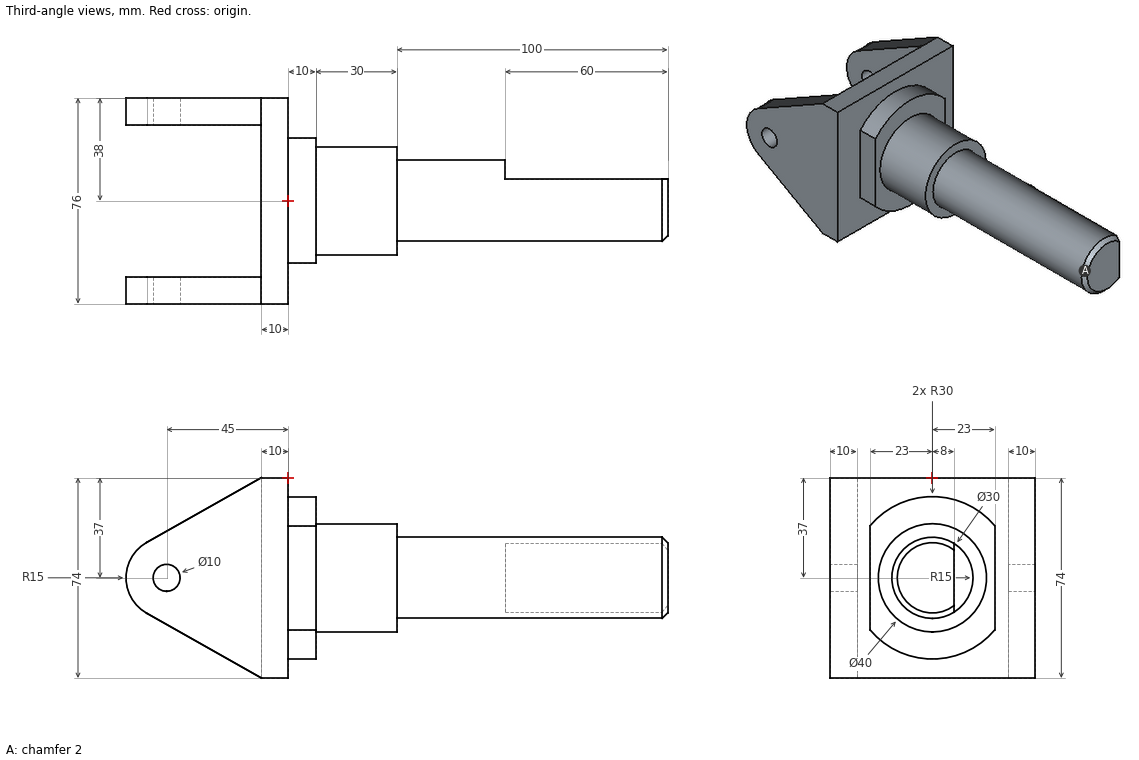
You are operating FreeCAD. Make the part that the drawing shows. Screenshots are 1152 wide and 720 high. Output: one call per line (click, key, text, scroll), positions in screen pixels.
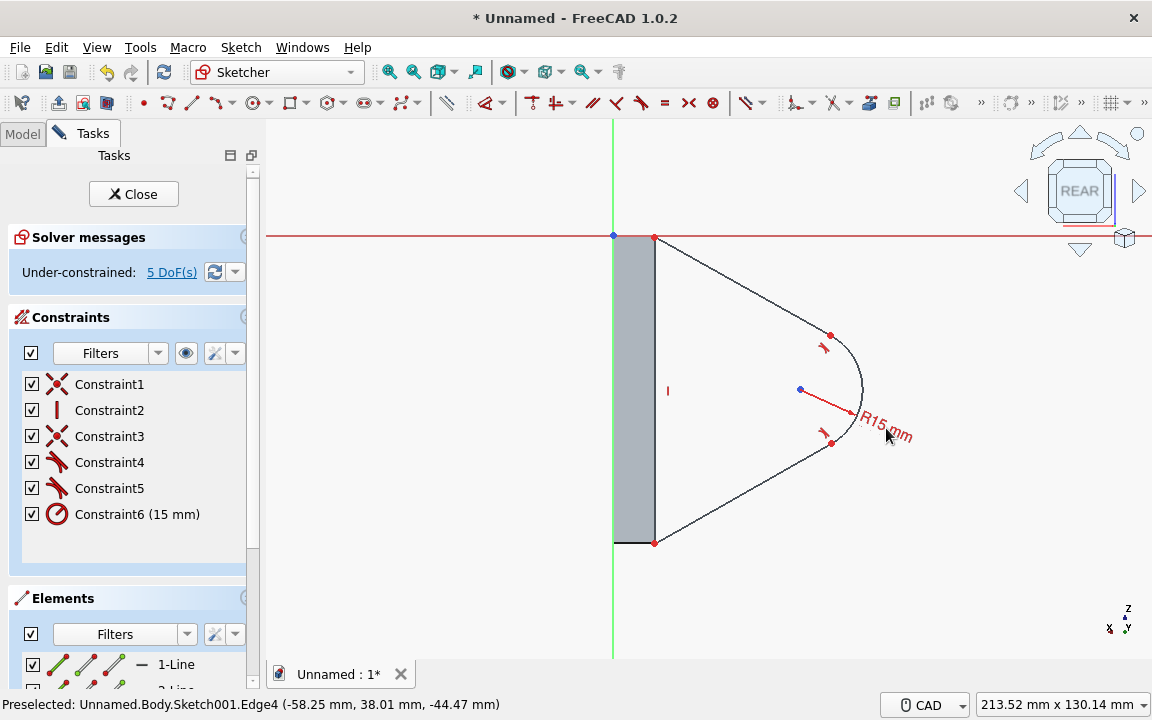
click(655, 237)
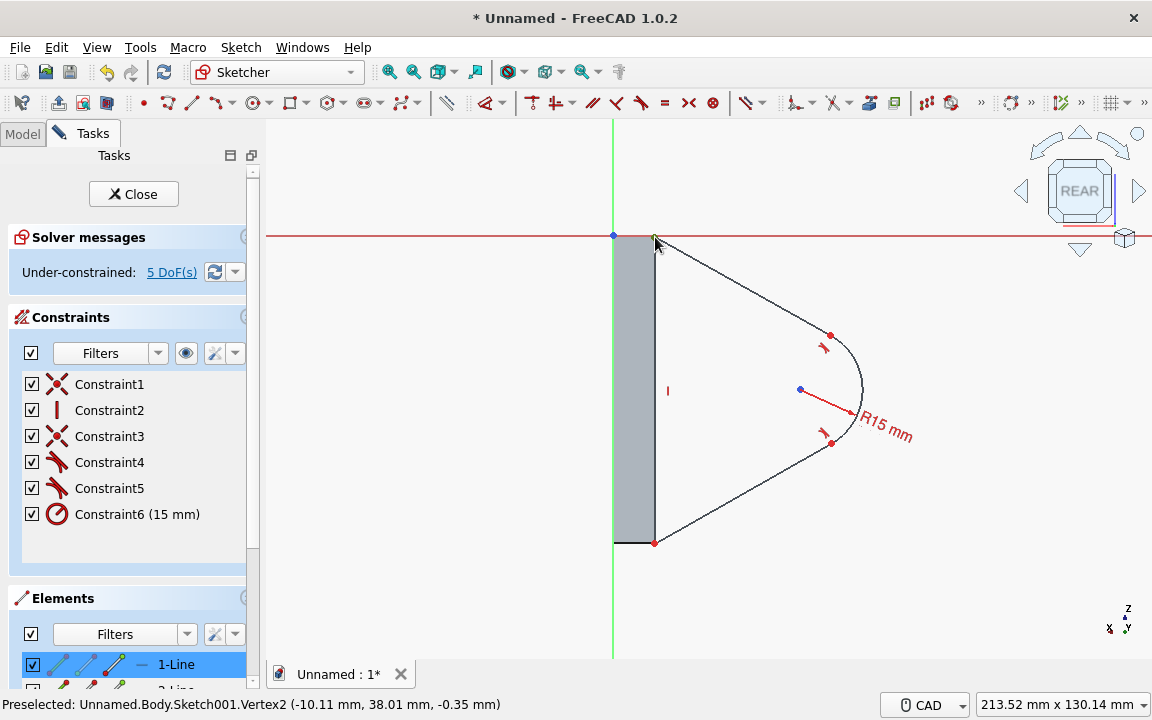
click(344, 236)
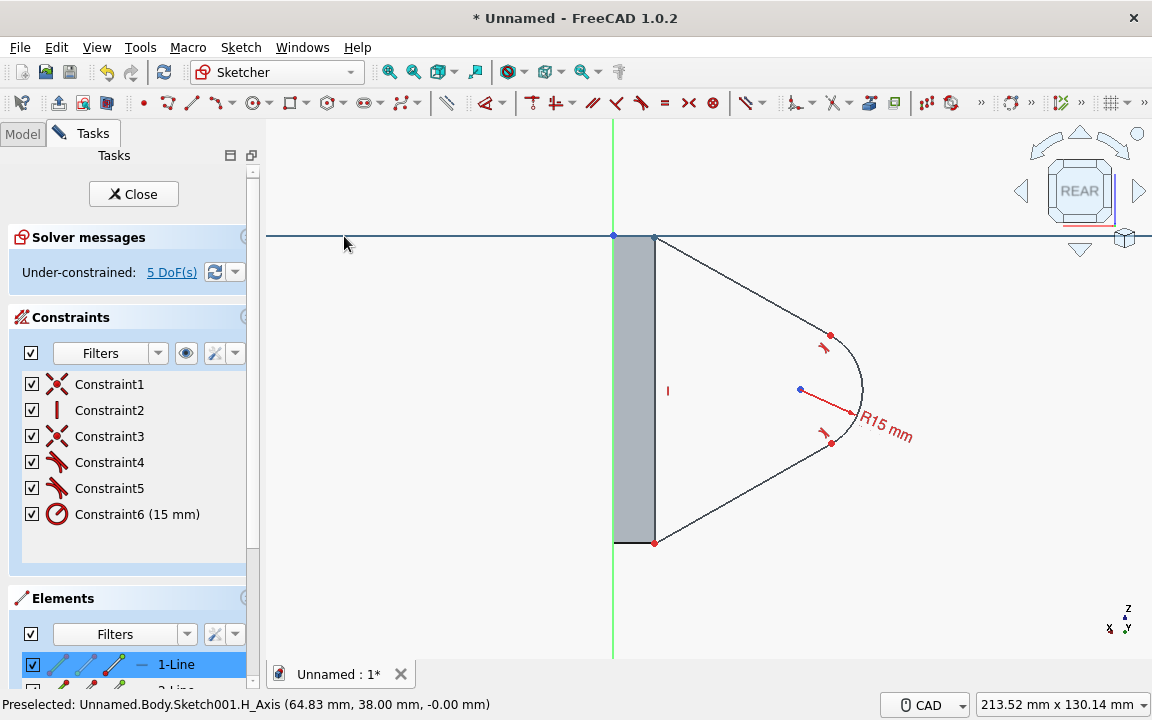
click(532, 104)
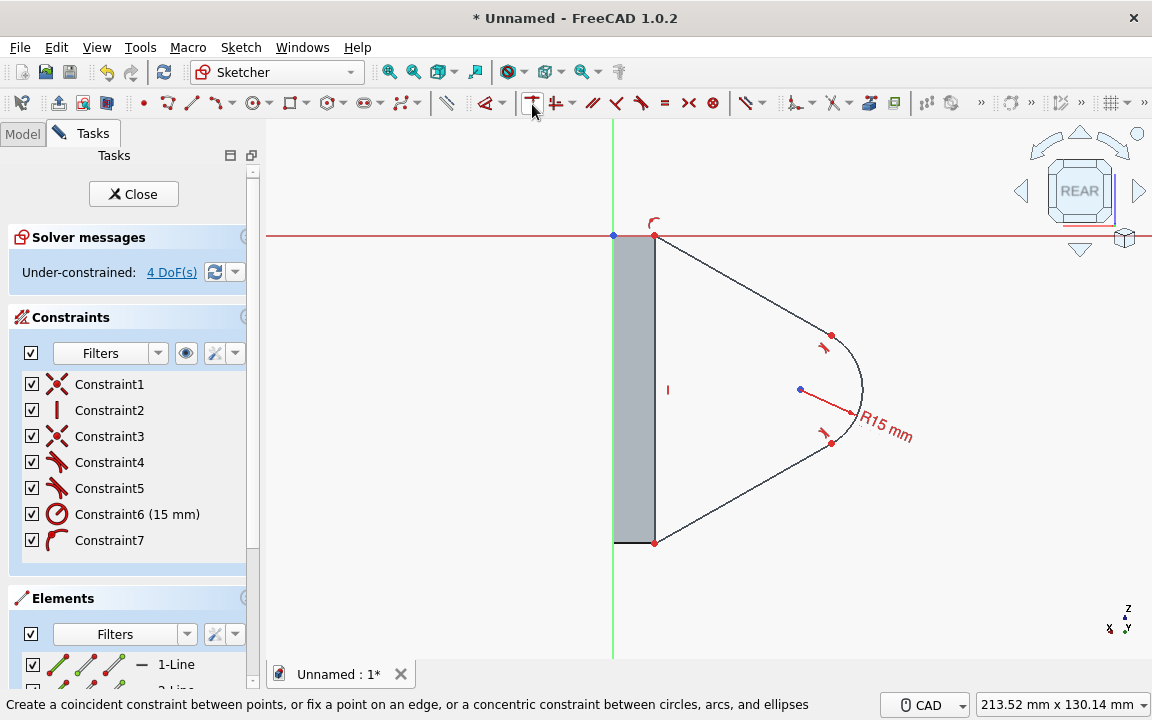
click(486, 104)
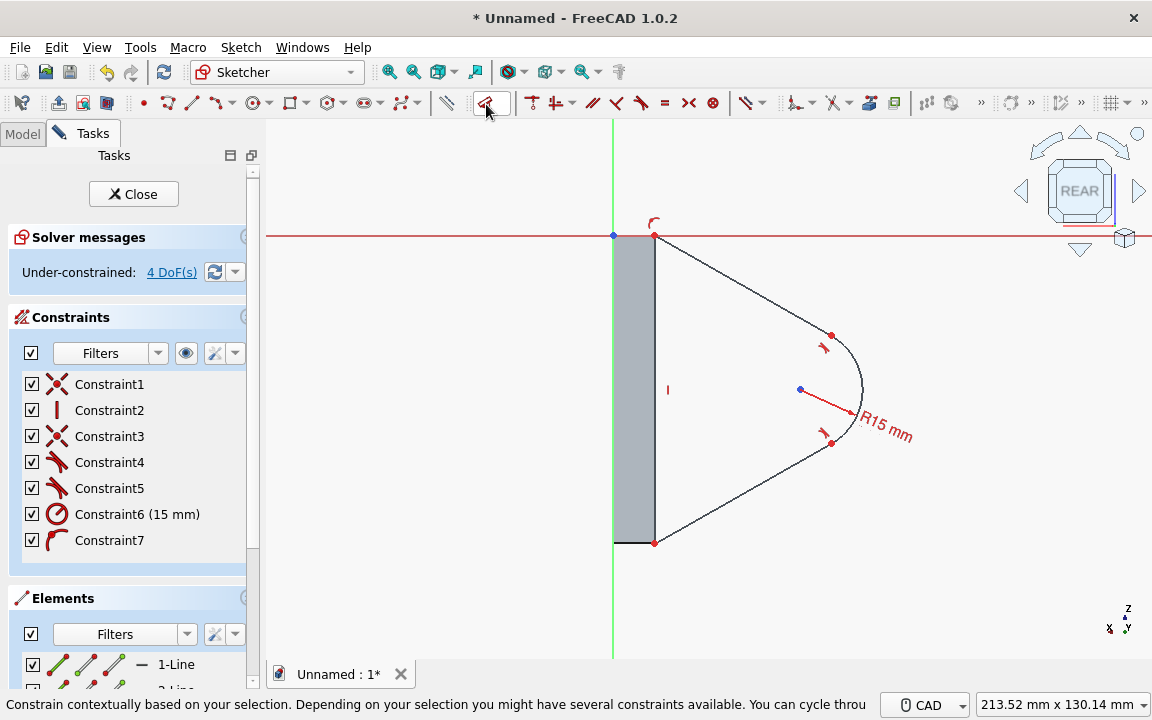
click(655, 328)
click(689, 390)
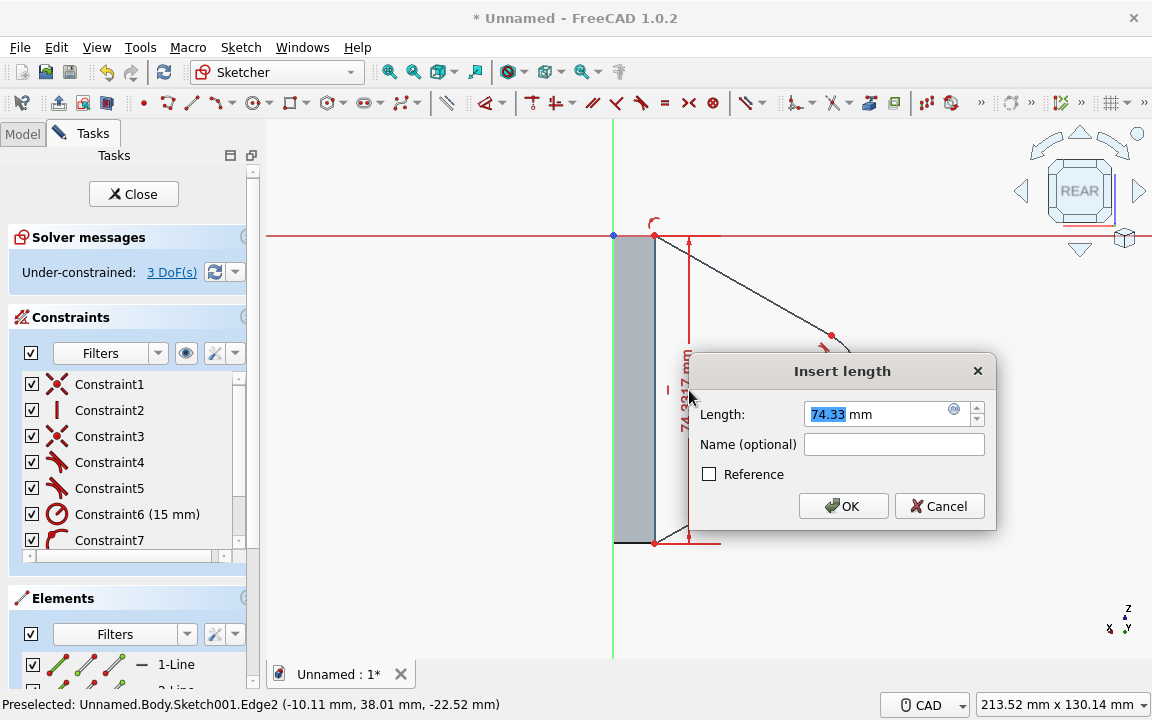
text(74)
key(Return)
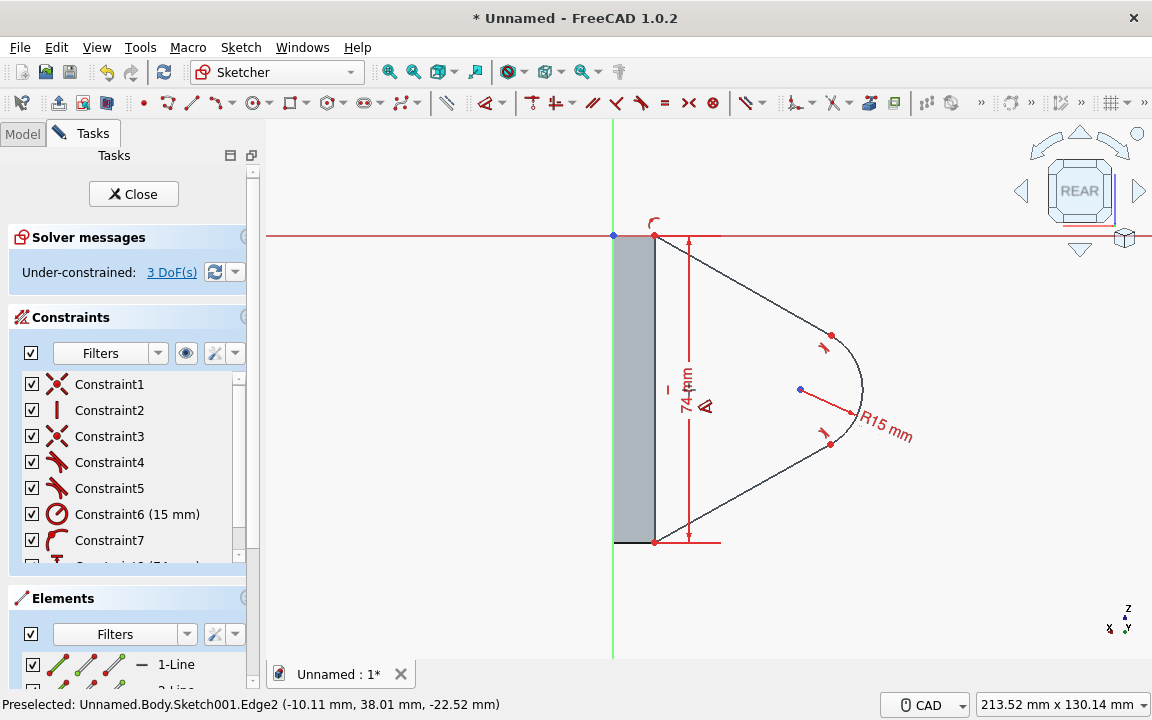
click(655, 236)
click(634, 202)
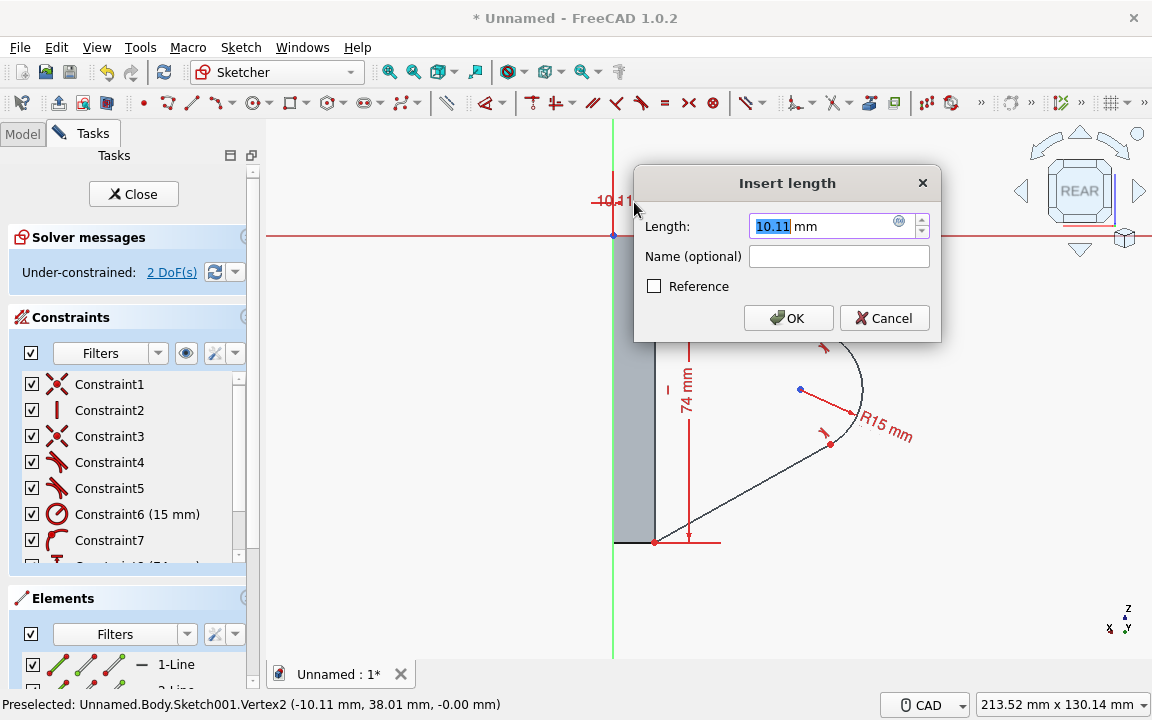
text(10)
key(Return)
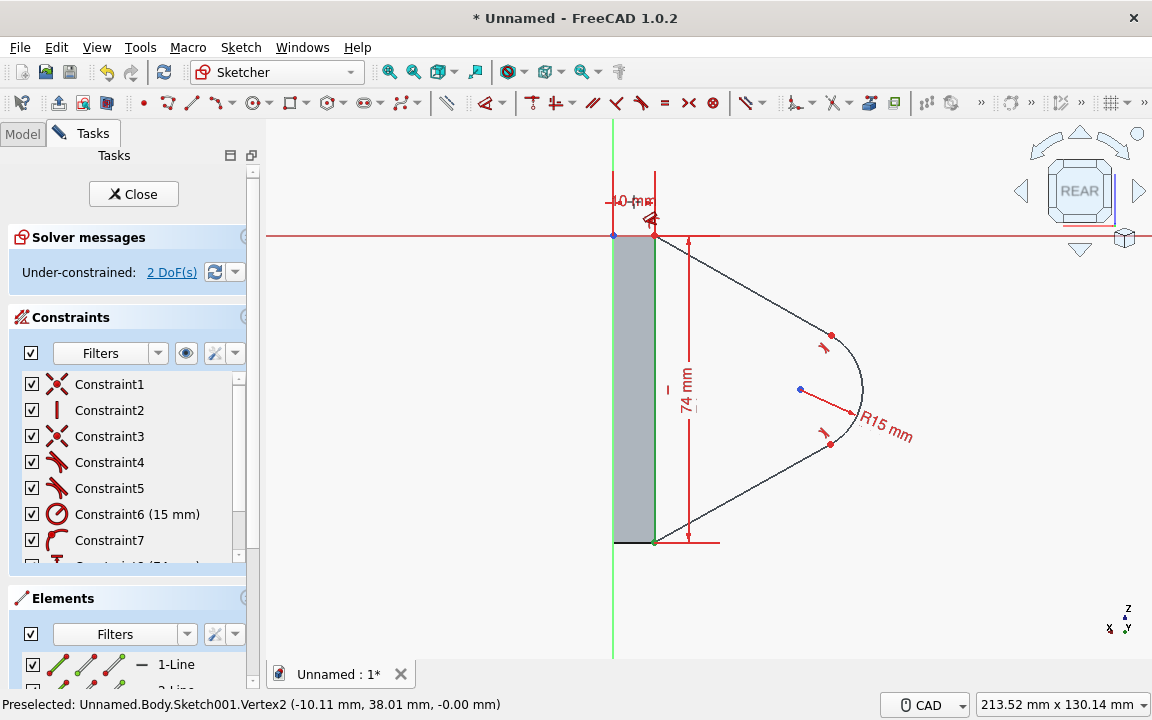
click(800, 390)
click(707, 202)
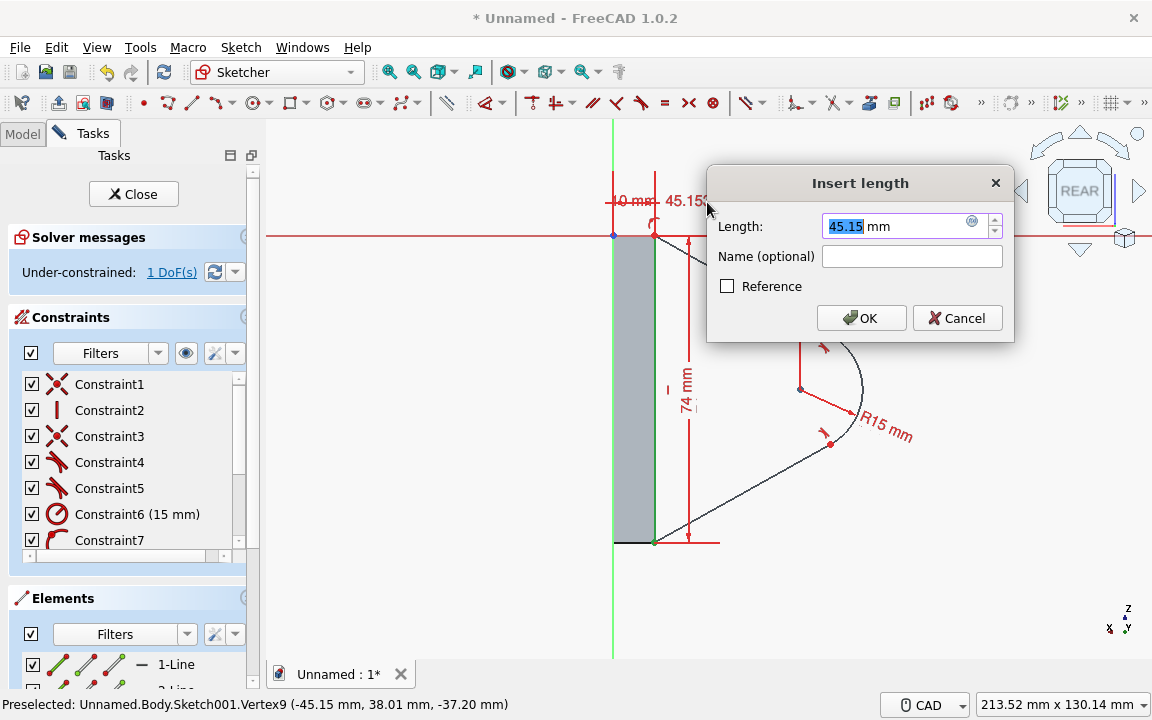
text(45)
key(Return)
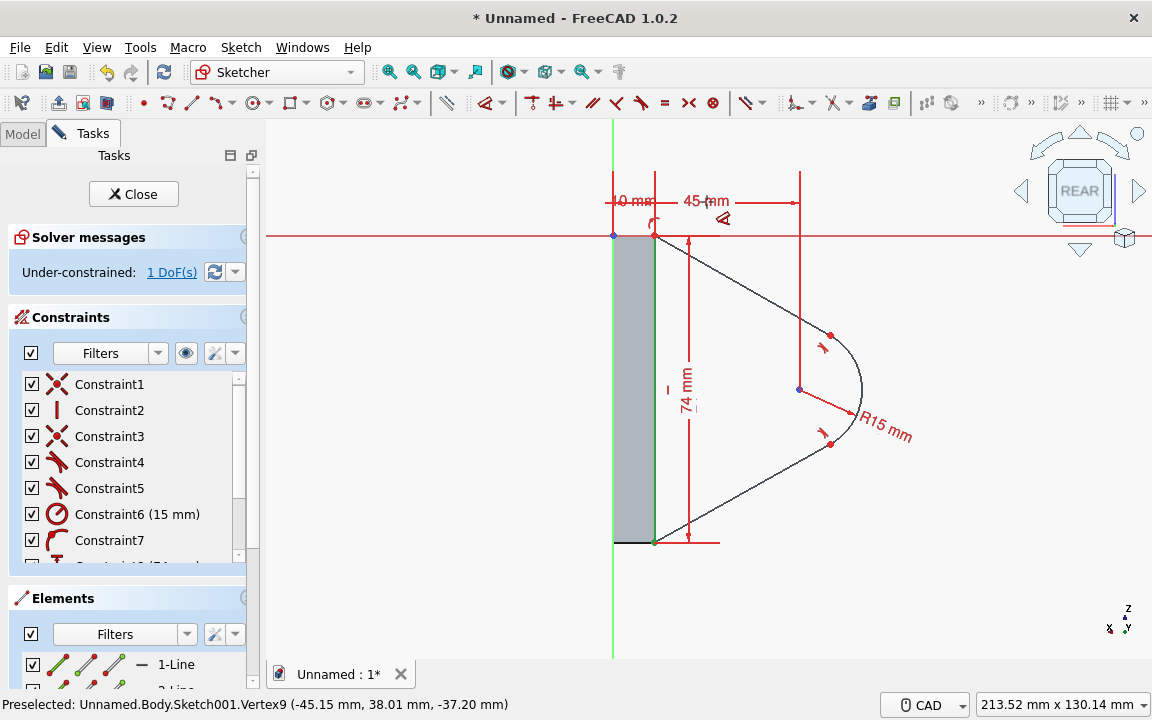
click(800, 390)
click(579, 313)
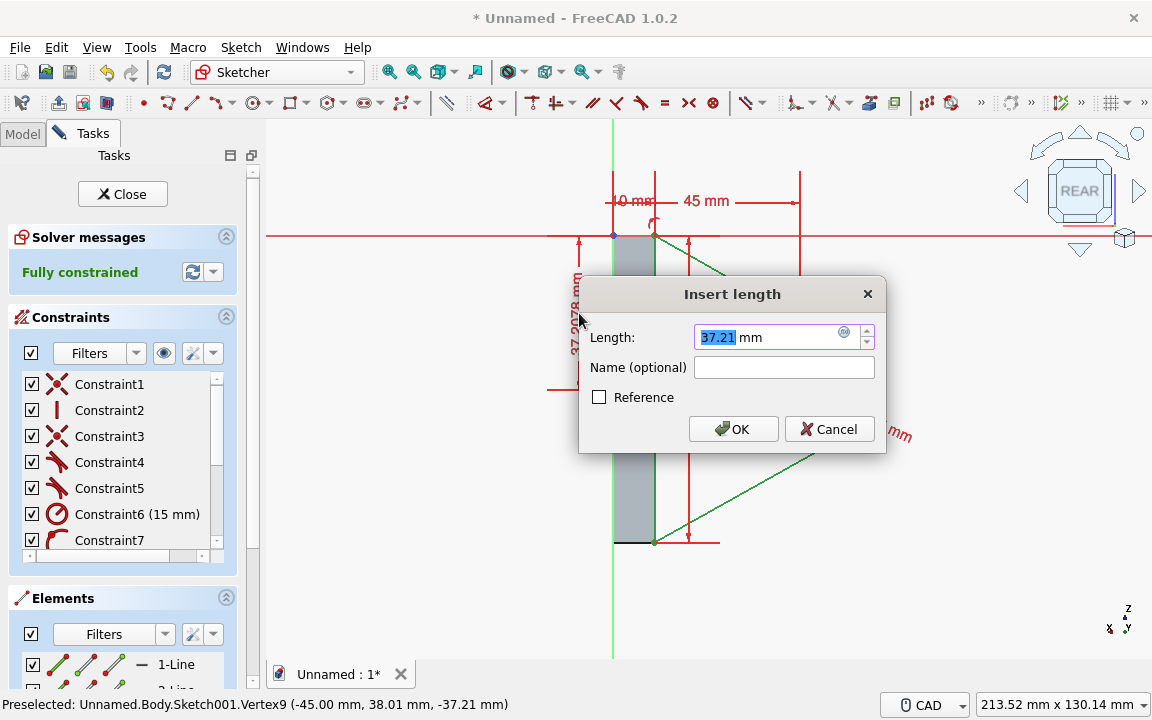
text(37)
key(Return)
key(Escape)